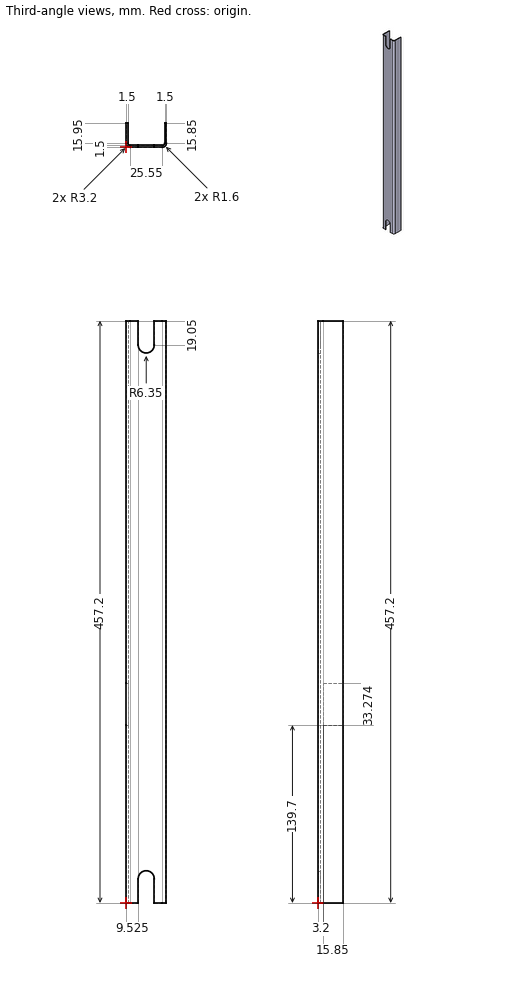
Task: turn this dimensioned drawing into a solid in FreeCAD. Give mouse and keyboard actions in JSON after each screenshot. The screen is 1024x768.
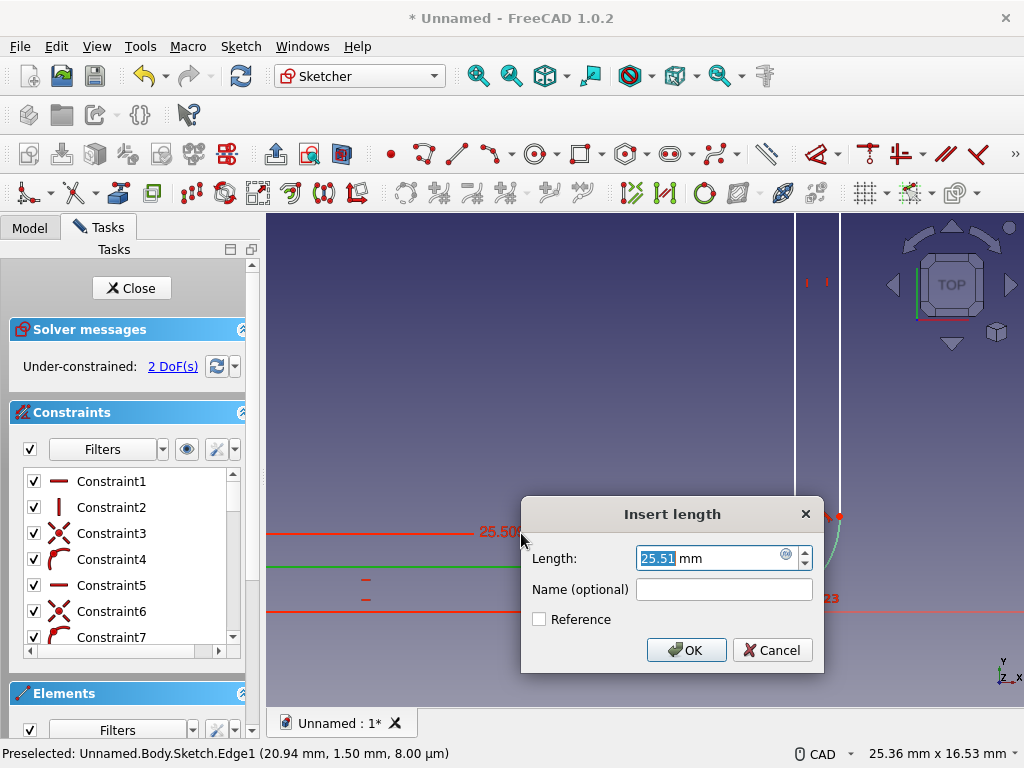
{"action": "type", "text": "25.55"}
{"action": "key", "text": "Return"}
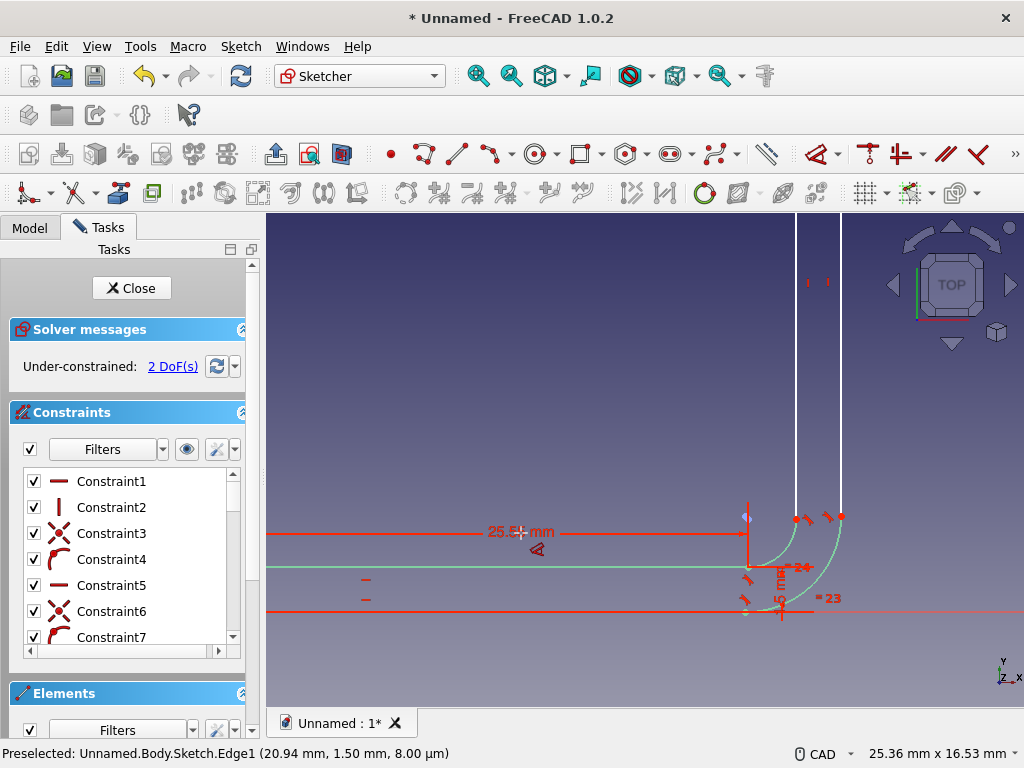
{"action": "scroll", "coordinate": [748, 568], "scroll_direction": "down", "scroll_amount": 4}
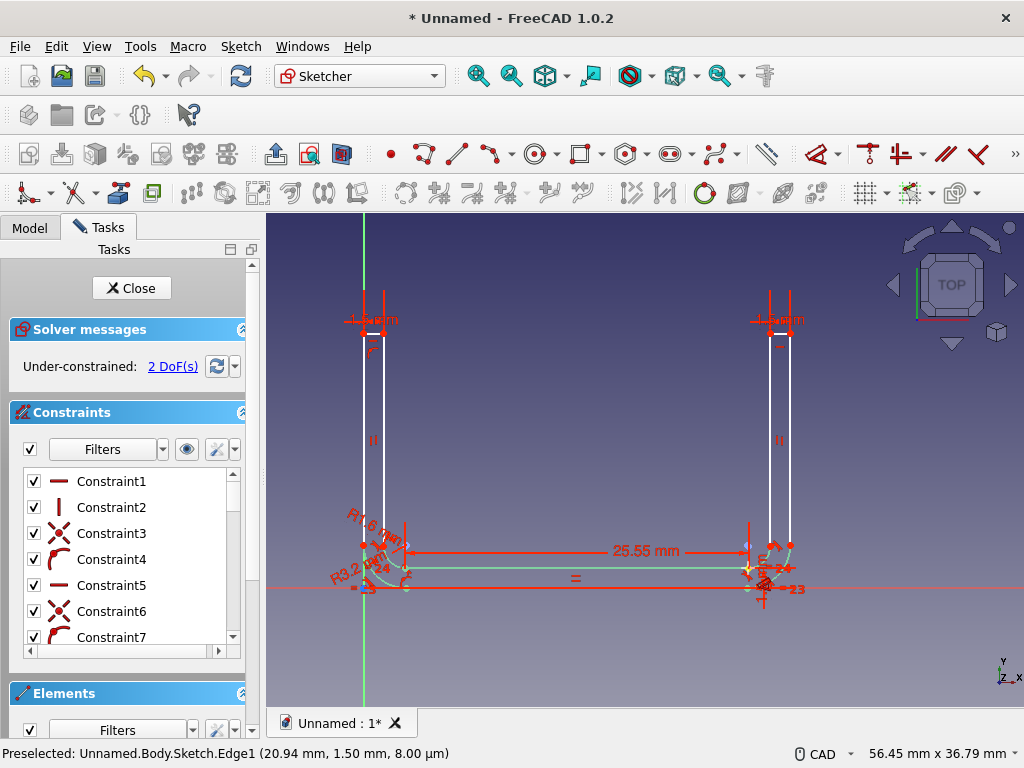
{"action": "left_click", "coordinate": [384, 483]}
{"action": "left_click", "coordinate": [350, 440]}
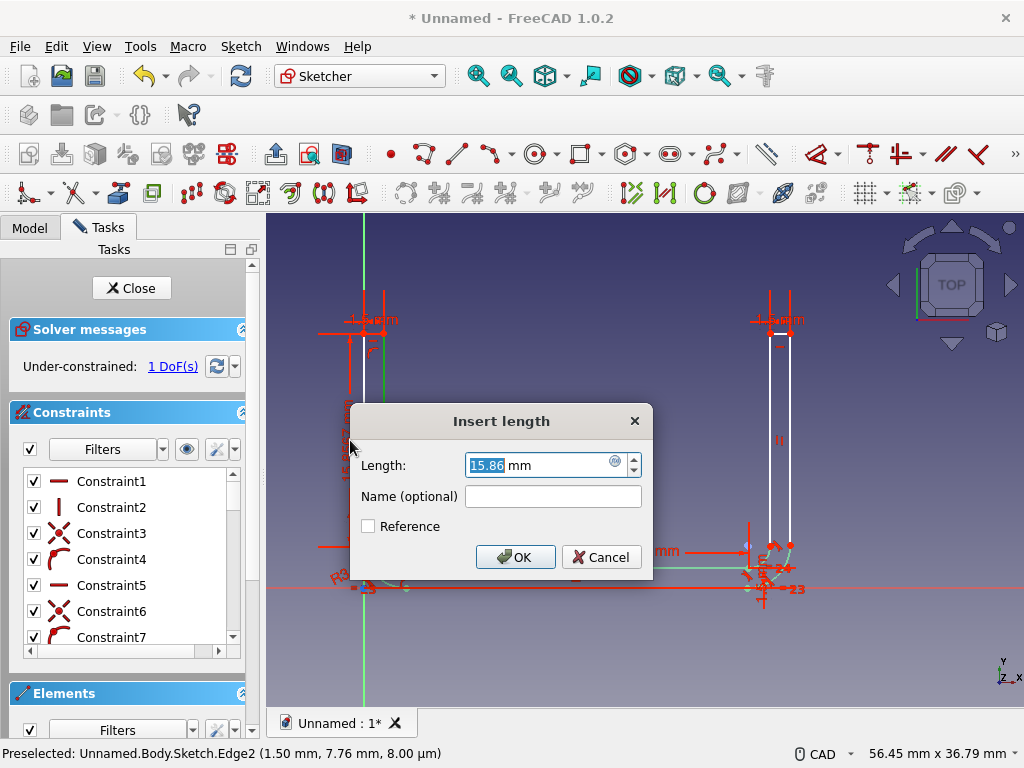
{"action": "type", "text": "15.95"}
{"action": "key", "text": "Return"}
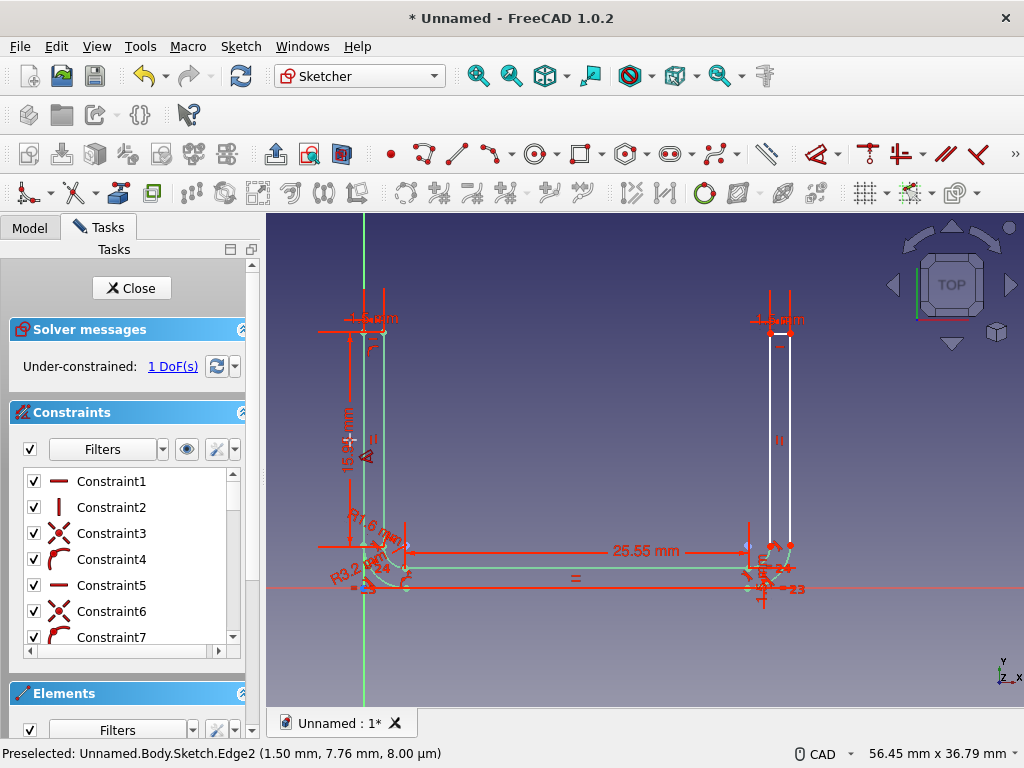
{"action": "left_click", "coordinate": [790, 482]}
{"action": "left_click", "coordinate": [824, 439]}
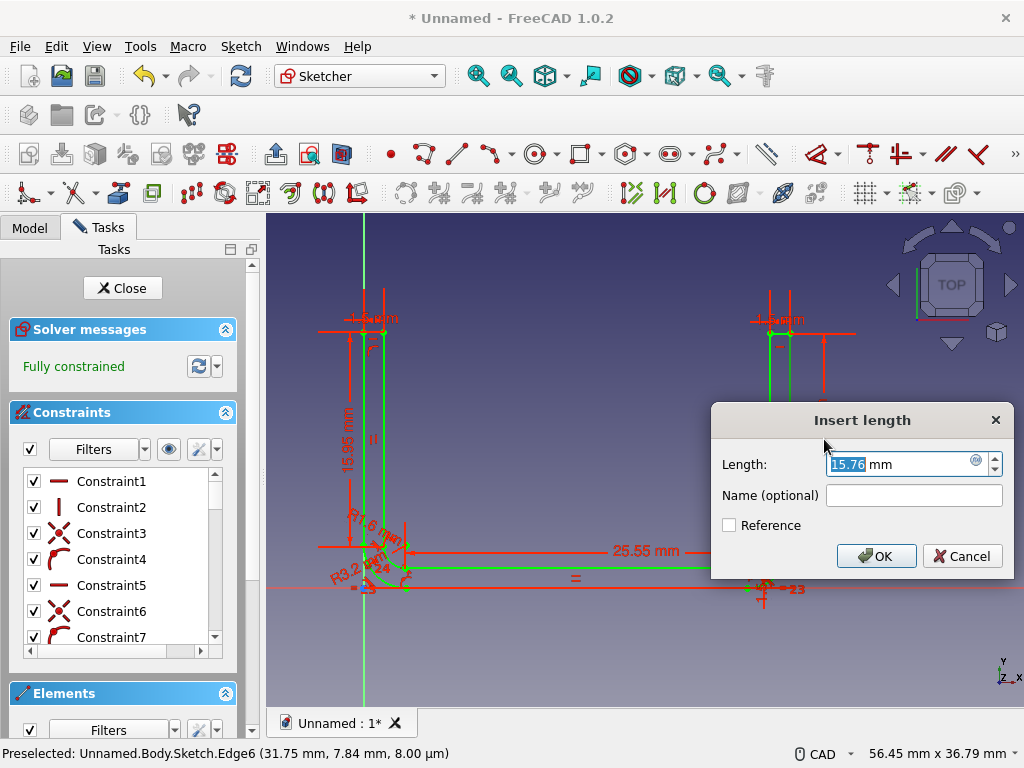
{"action": "type", "text": "15.85"}
{"action": "key", "text": "Return"}
{"action": "key", "text": "Escape"}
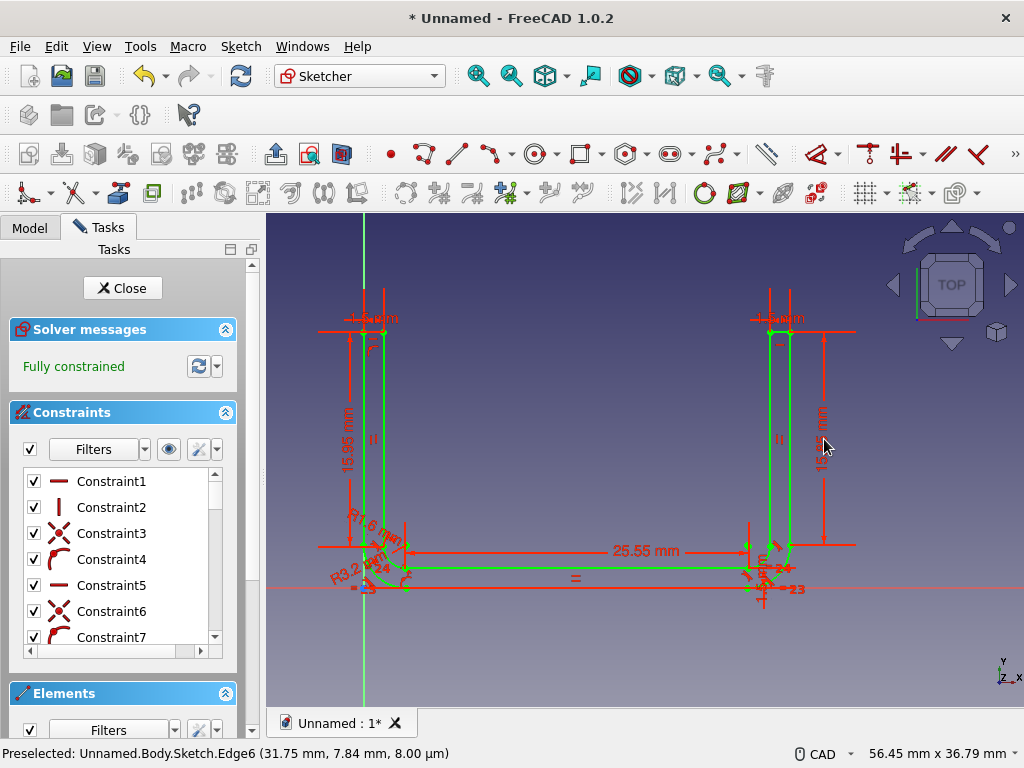
{"action": "left_click", "coordinate": [123, 288]}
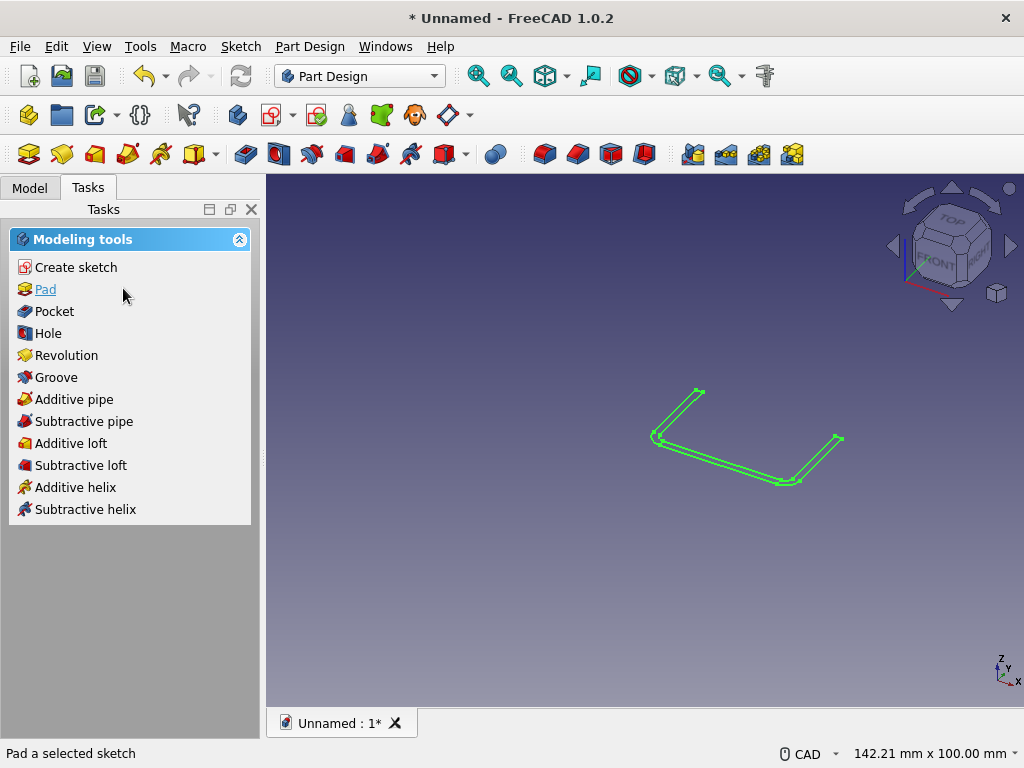
{"action": "left_click", "coordinate": [29, 154]}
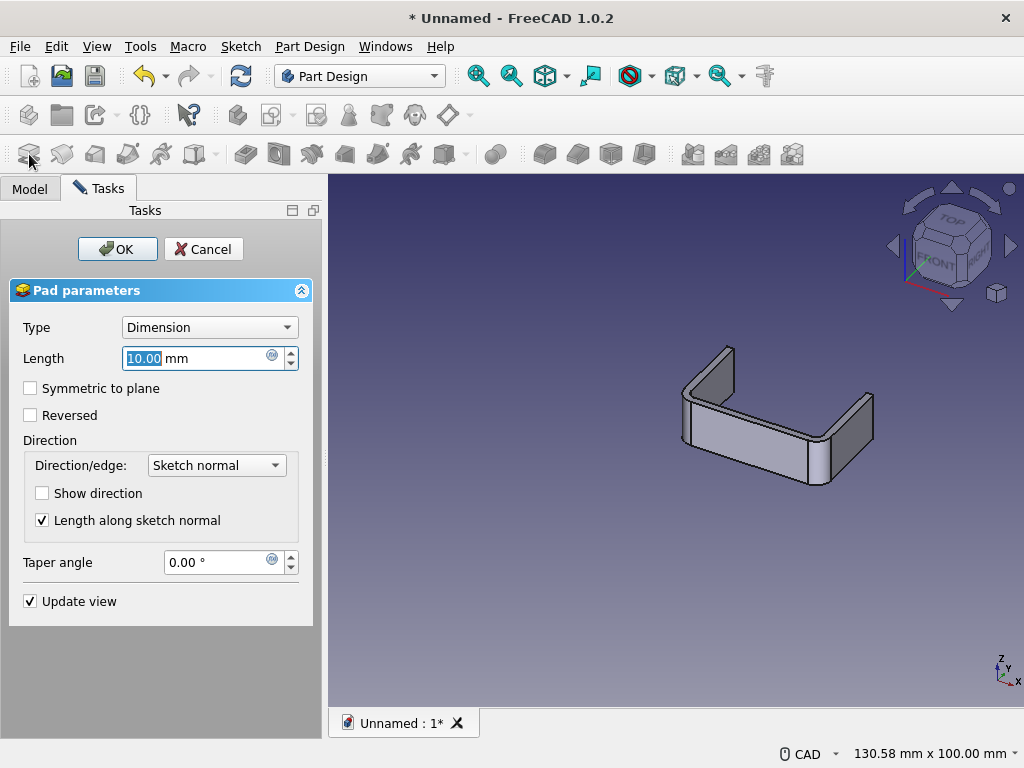
{"action": "type", "text": "457.2"}
{"action": "key", "text": "Tab"}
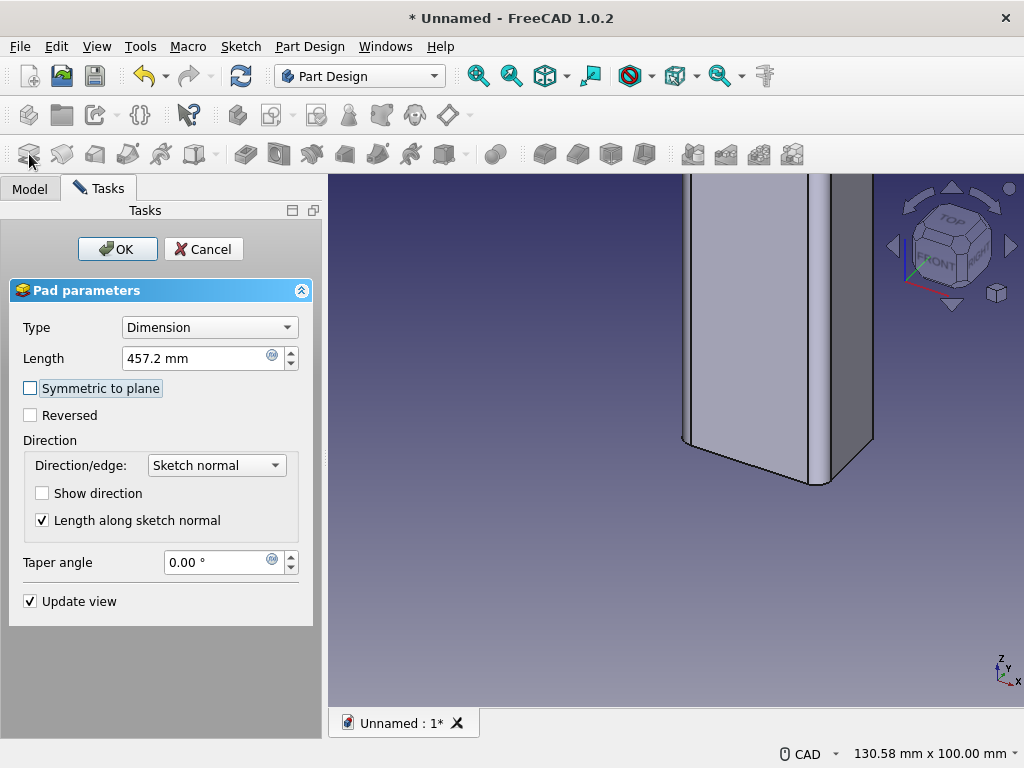
{"action": "left_click", "coordinate": [118, 249]}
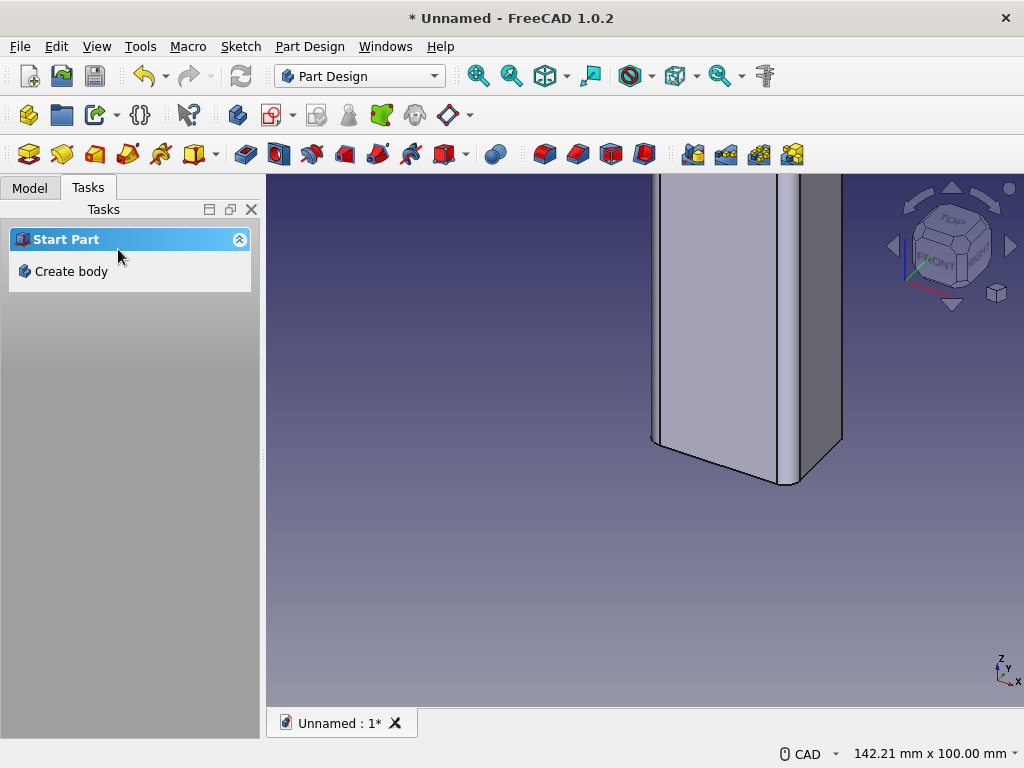
{"action": "key", "text": "v f"}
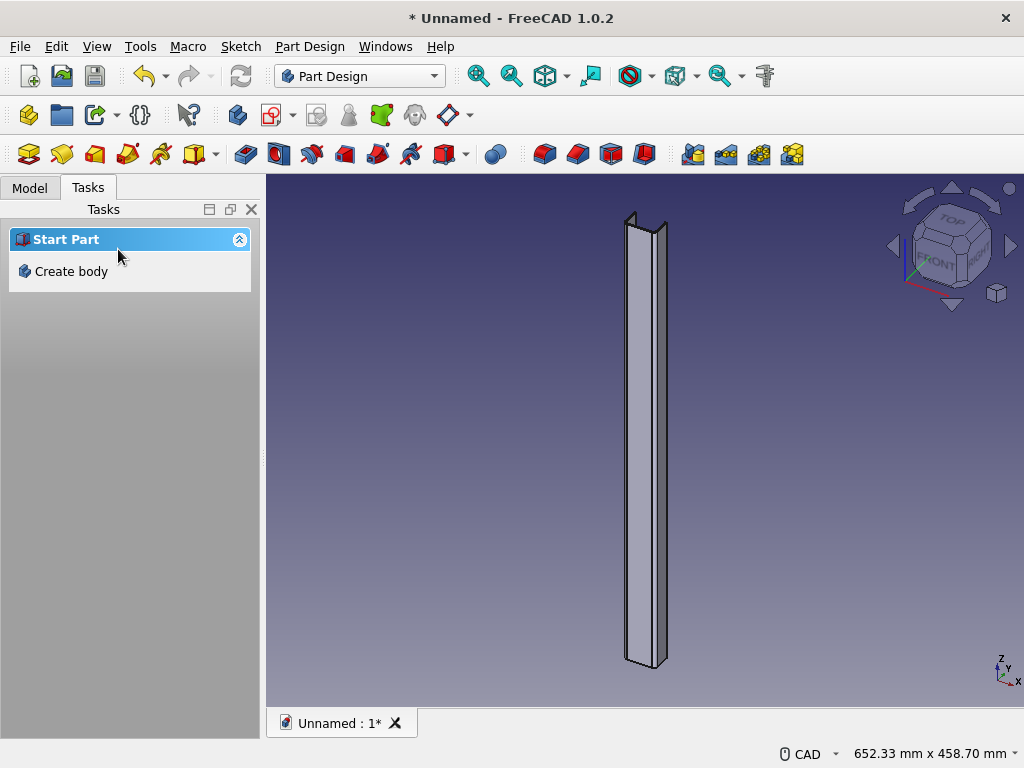
{"action": "key", "text": "6"}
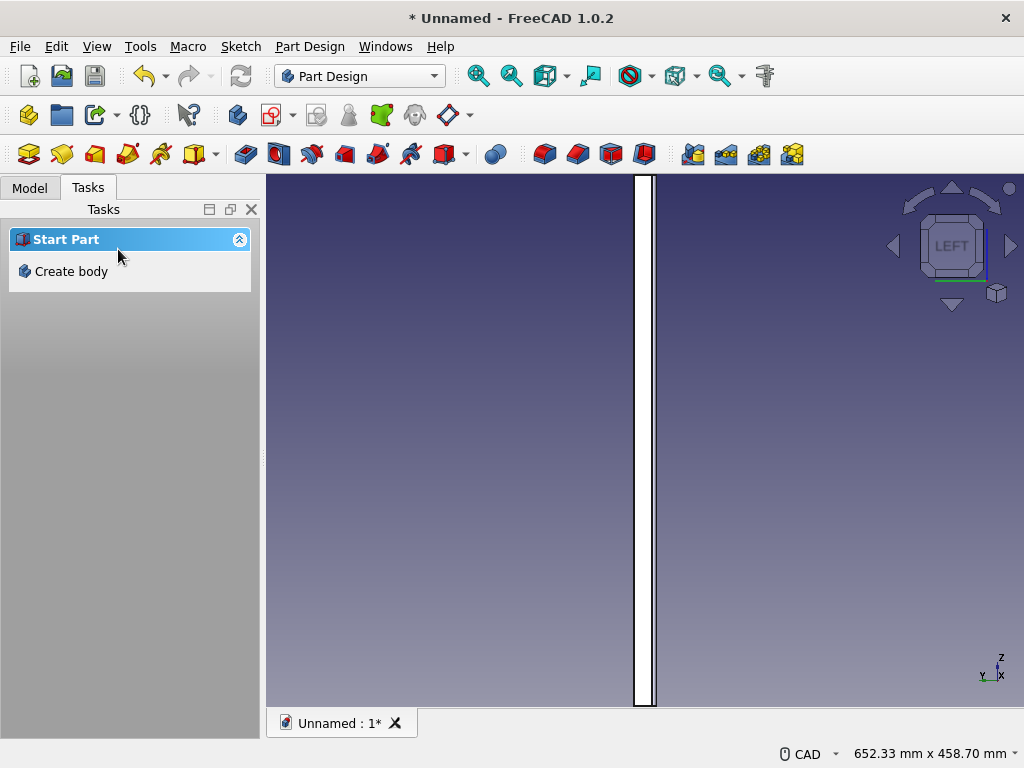
{"action": "left_click", "coordinate": [643, 212]}